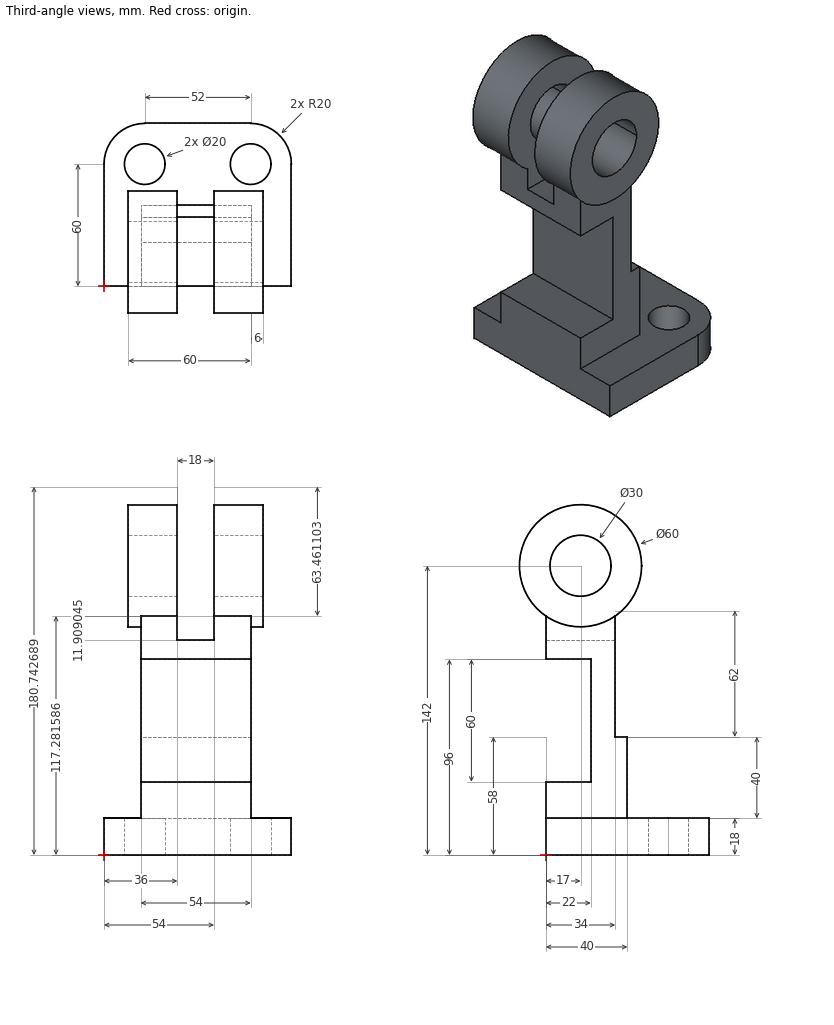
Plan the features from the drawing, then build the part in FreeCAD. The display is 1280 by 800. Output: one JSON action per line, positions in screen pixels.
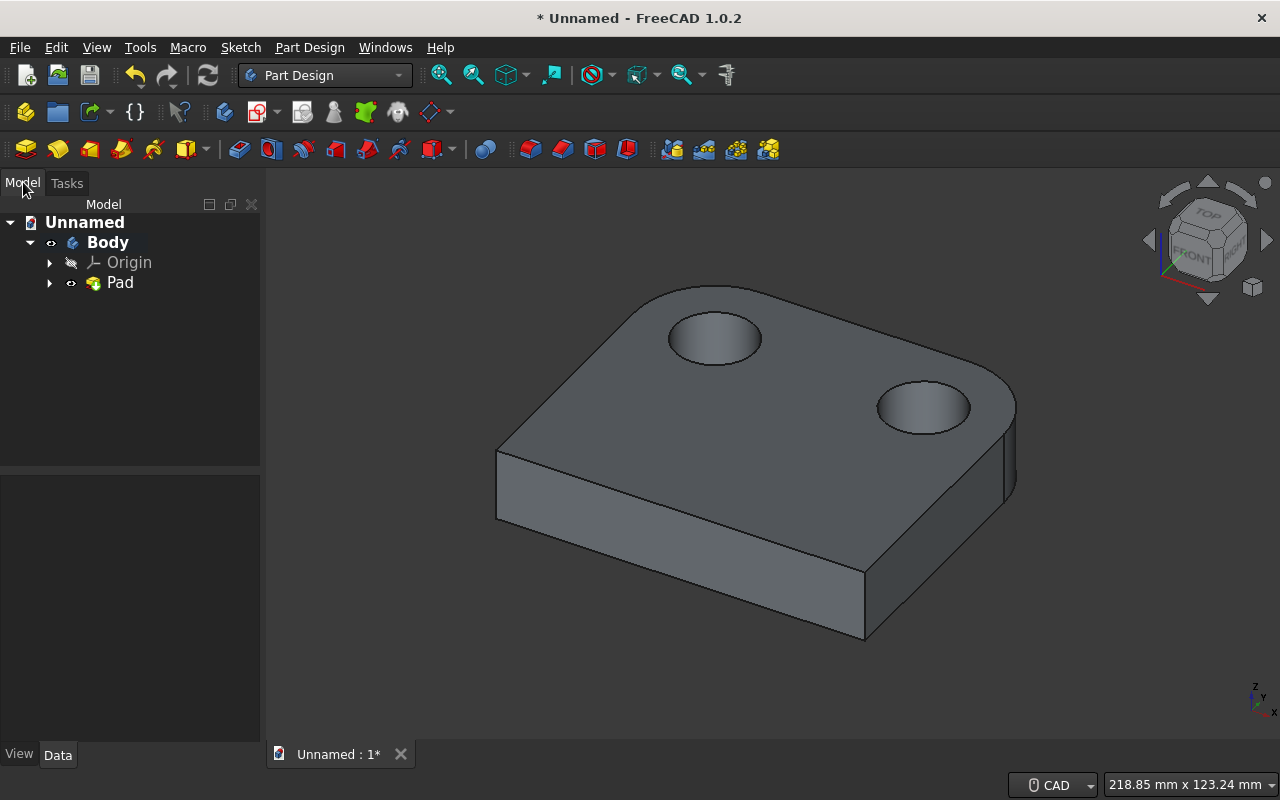
{"action": "left_click", "coordinate": [50, 263]}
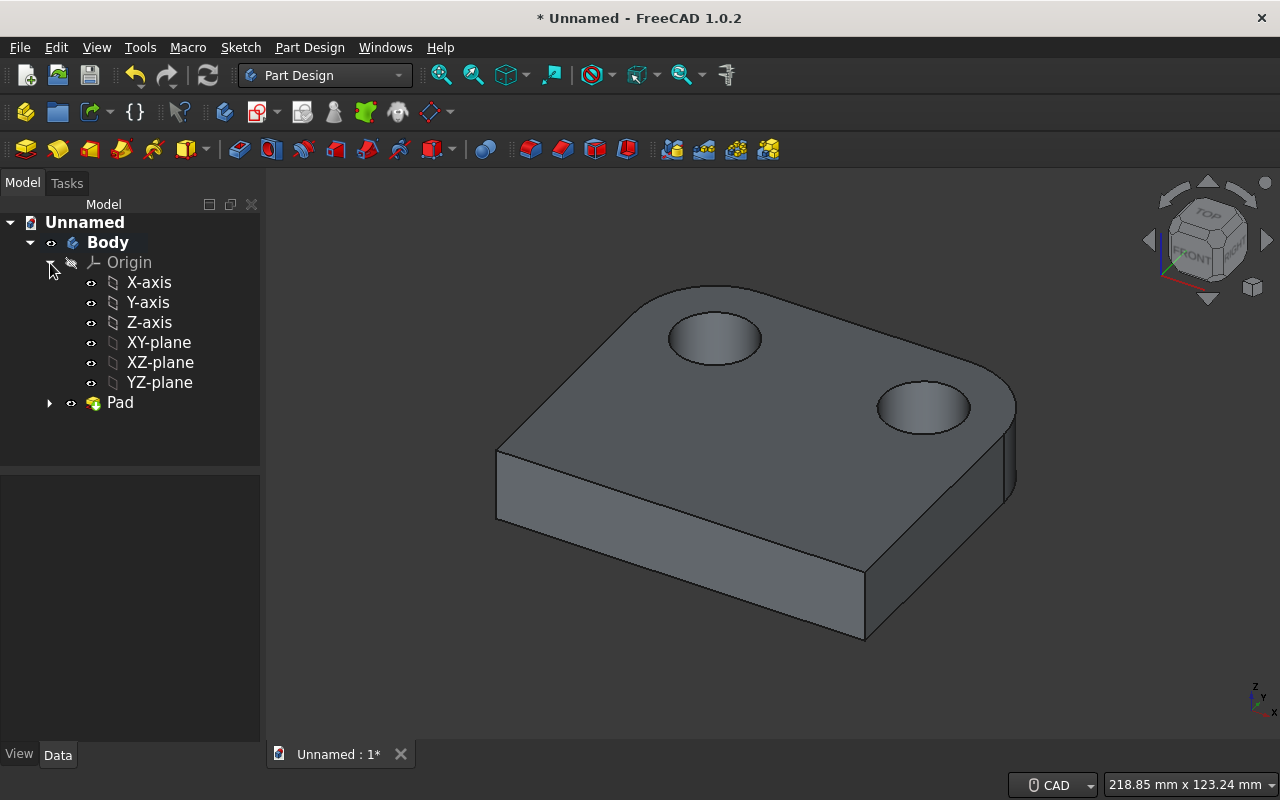
{"action": "left_click", "coordinate": [136, 383]}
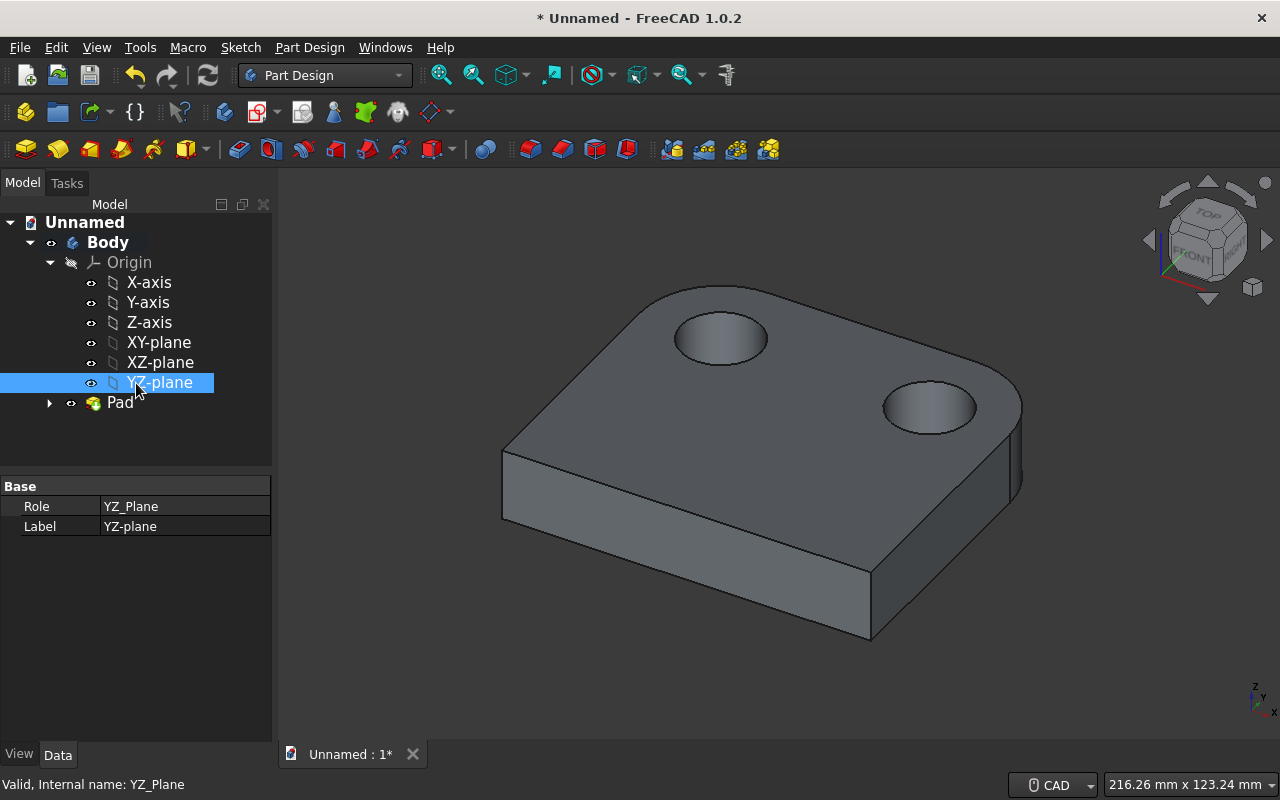
{"action": "left_click", "coordinate": [430, 112]}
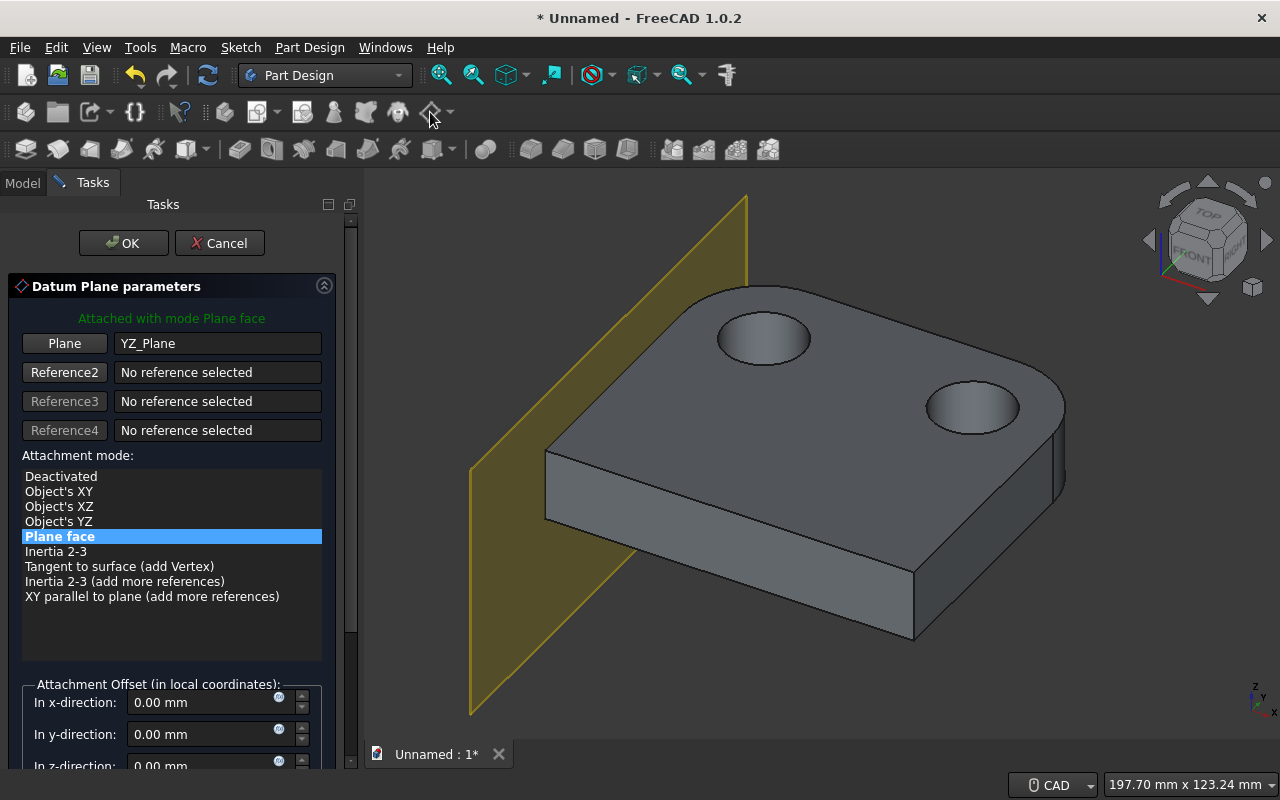
{"action": "scroll", "coordinate": [351, 491], "scroll_direction": "down", "scroll_amount": 2}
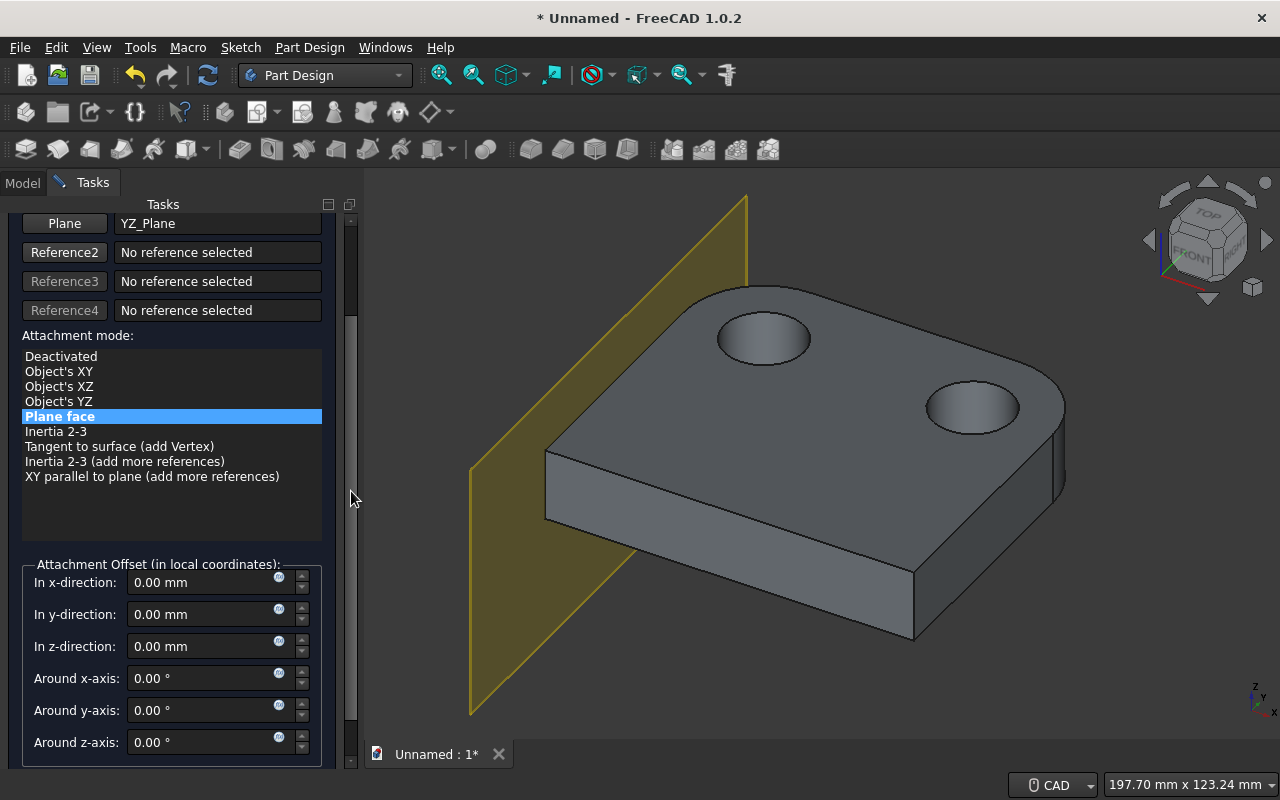
{"action": "triple_click", "coordinate": [210, 646]}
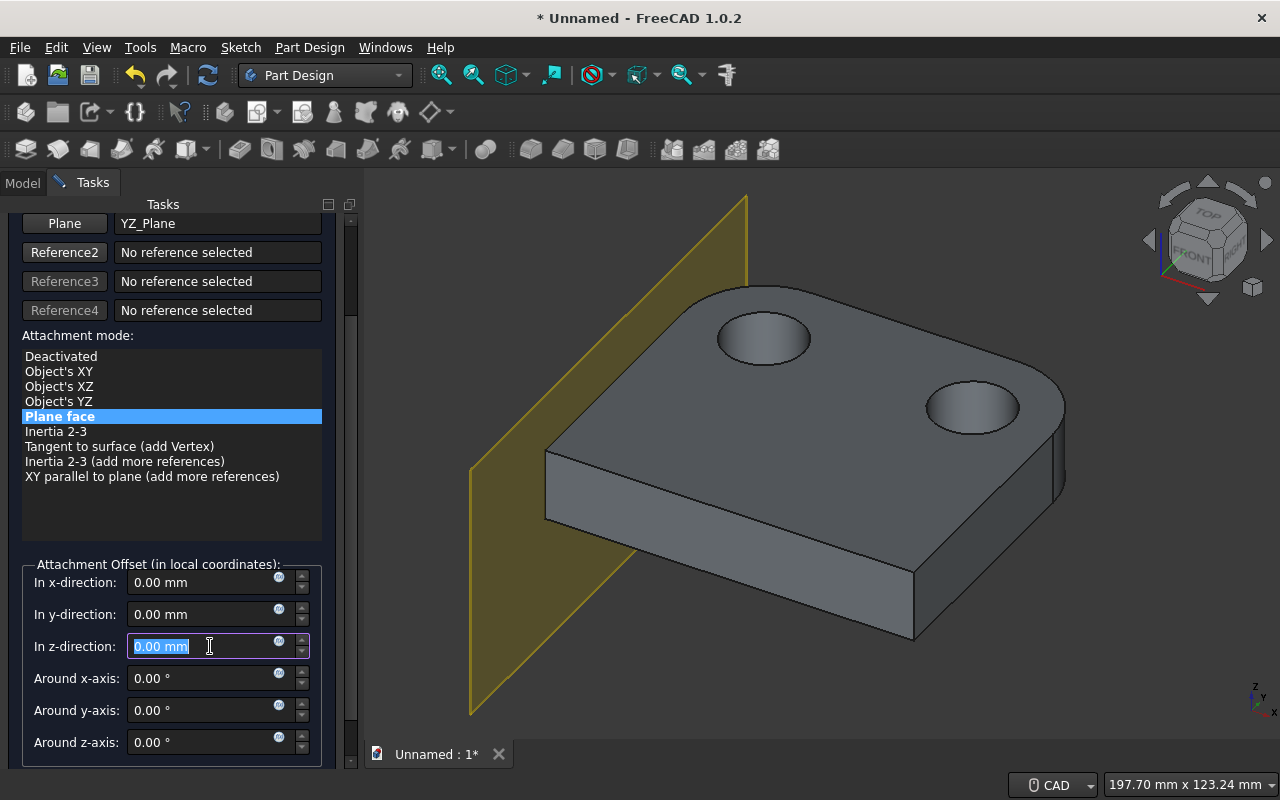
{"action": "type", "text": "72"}
{"action": "key", "text": "Tab"}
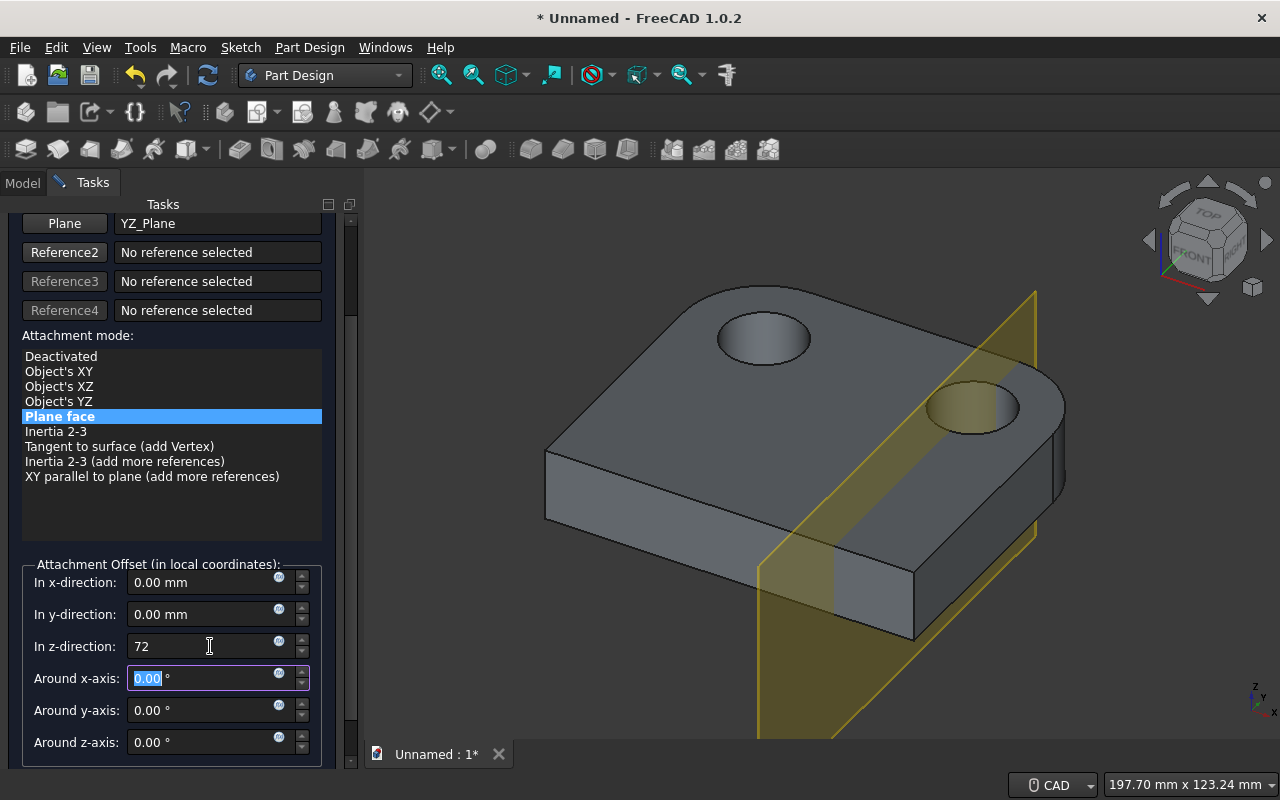
{"action": "scroll", "coordinate": [351, 491], "scroll_direction": "up", "scroll_amount": 3}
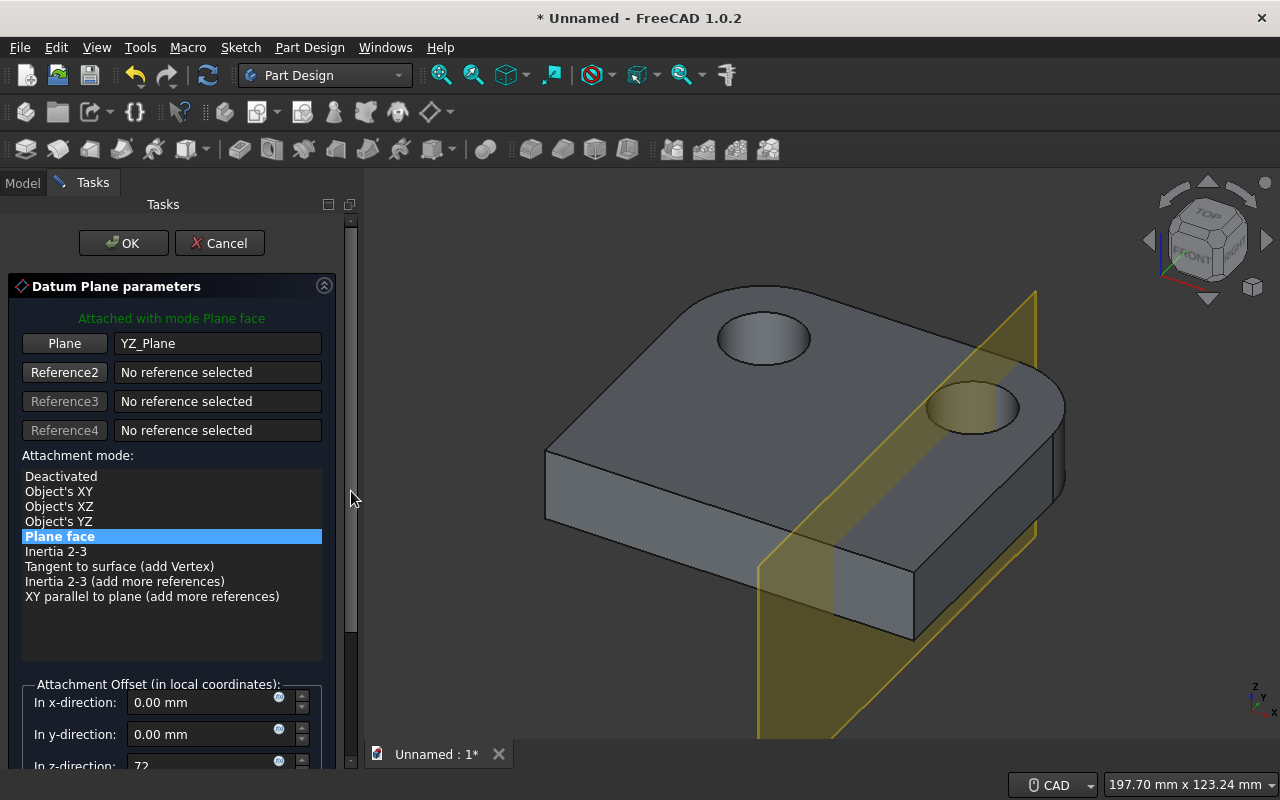
{"action": "left_click", "coordinate": [124, 243]}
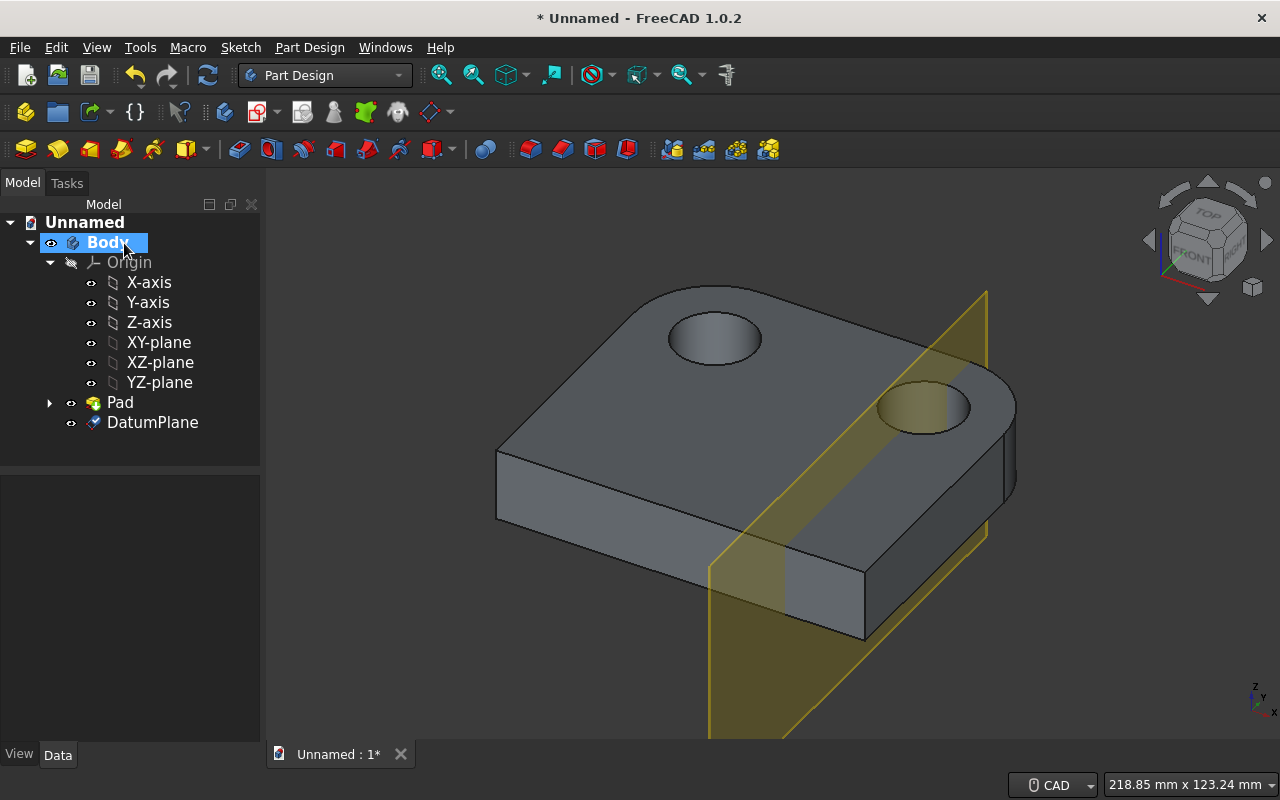
{"action": "left_click", "coordinate": [116, 423]}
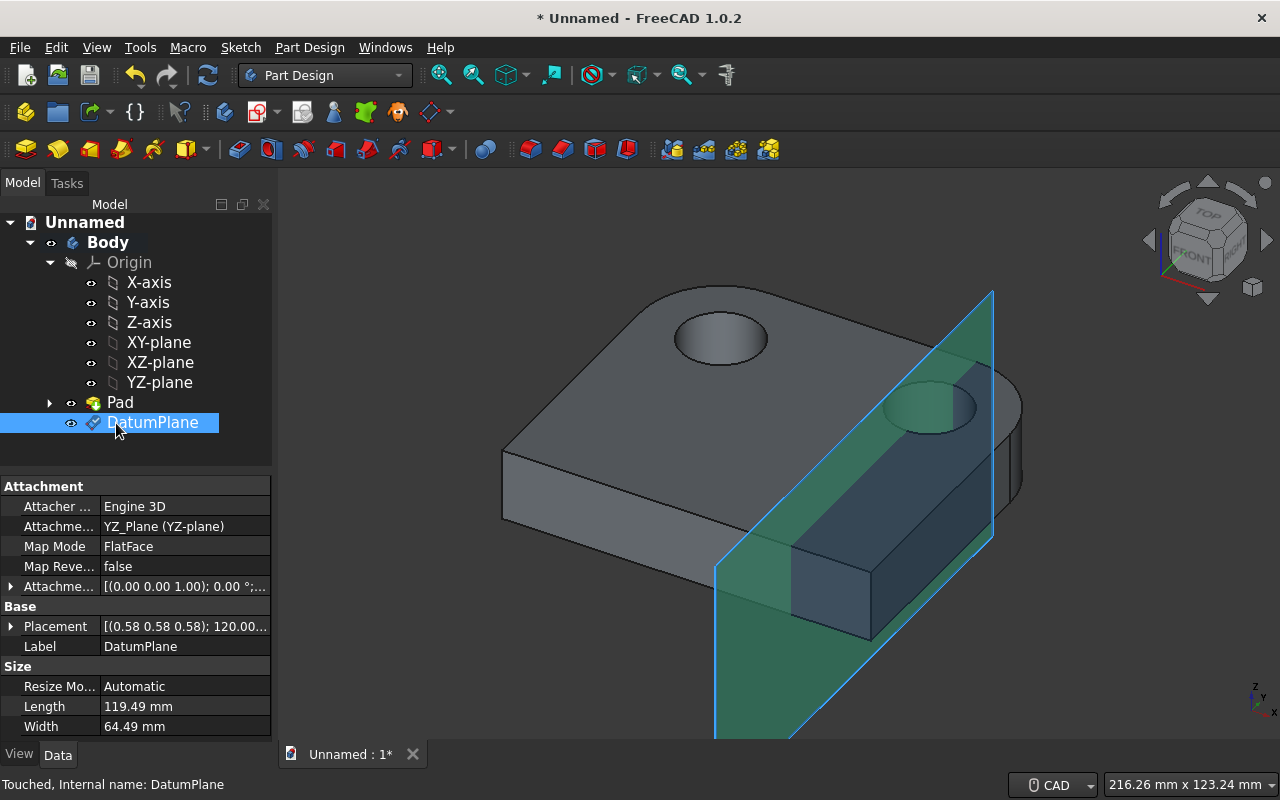
{"action": "left_click", "coordinate": [258, 112]}